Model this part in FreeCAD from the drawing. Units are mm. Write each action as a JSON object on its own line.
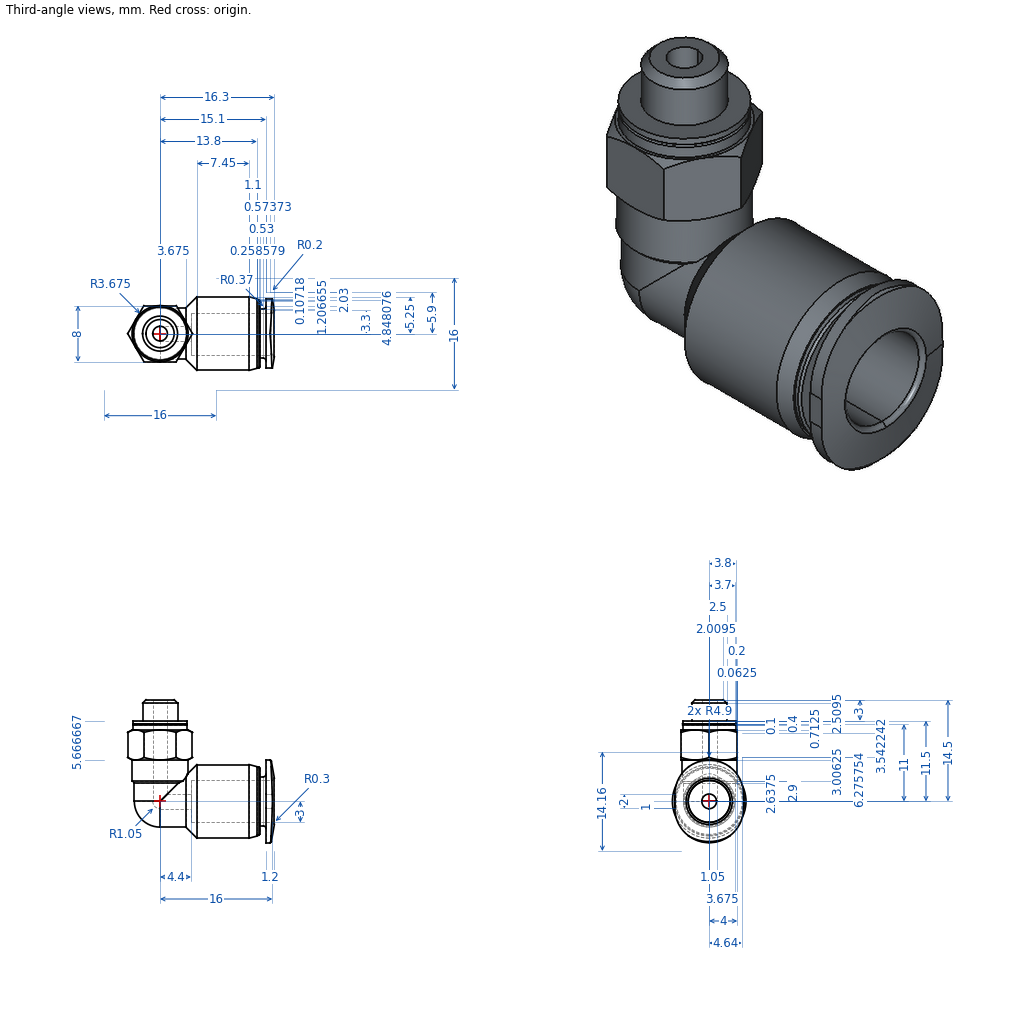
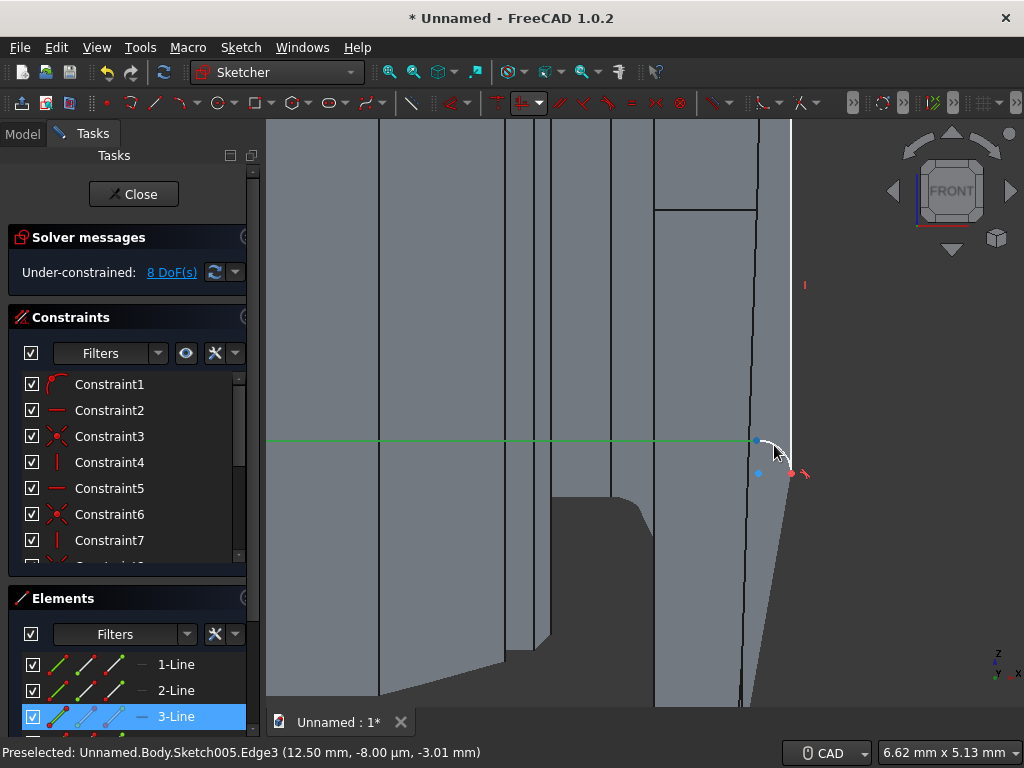
{"action": "left_click", "coordinate": [772, 443]}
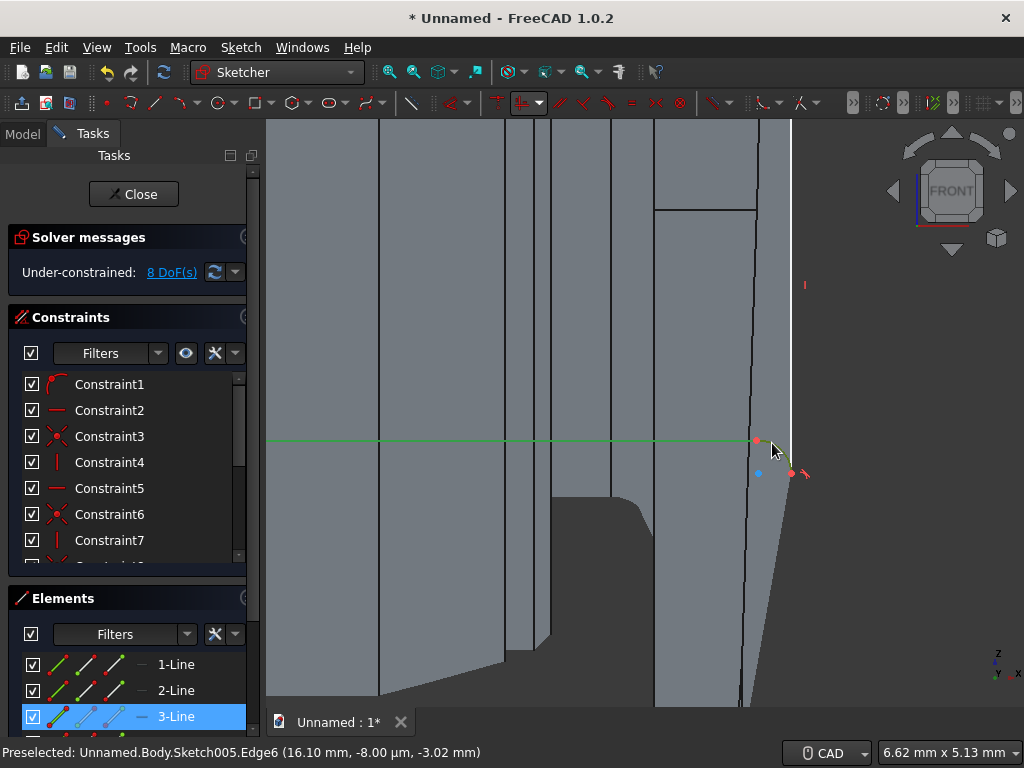
{"action": "left_click", "coordinate": [608, 104]}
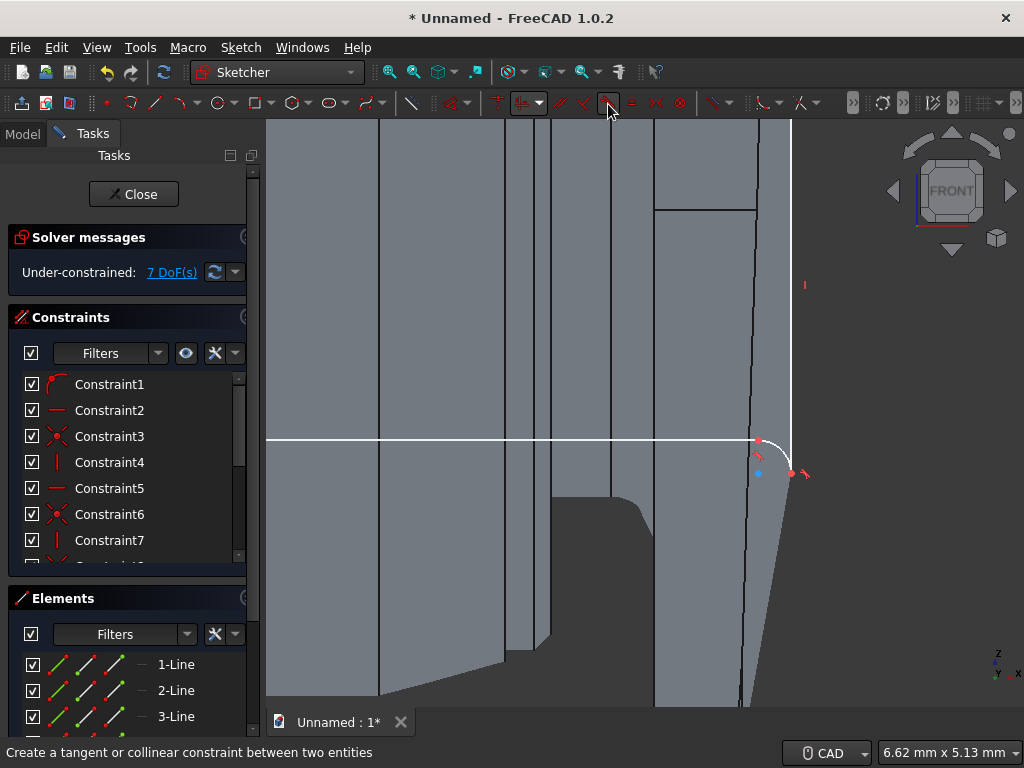
{"action": "scroll", "coordinate": [774, 445], "scroll_direction": "down", "scroll_amount": 8}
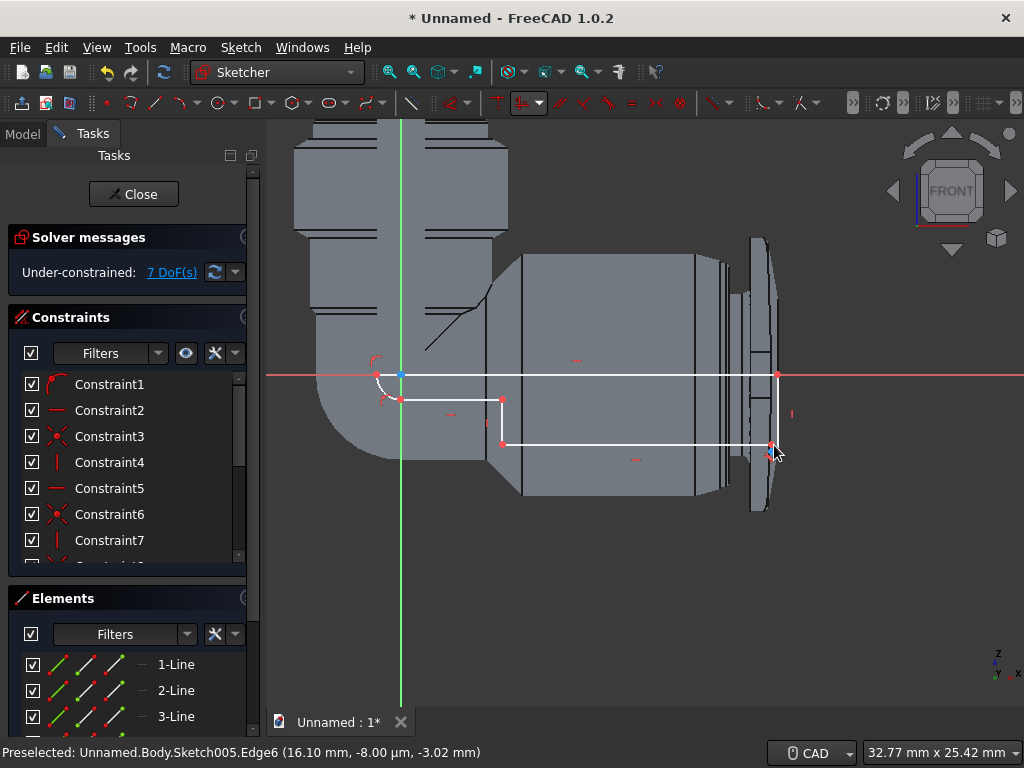
{"action": "left_click", "coordinate": [472, 400]}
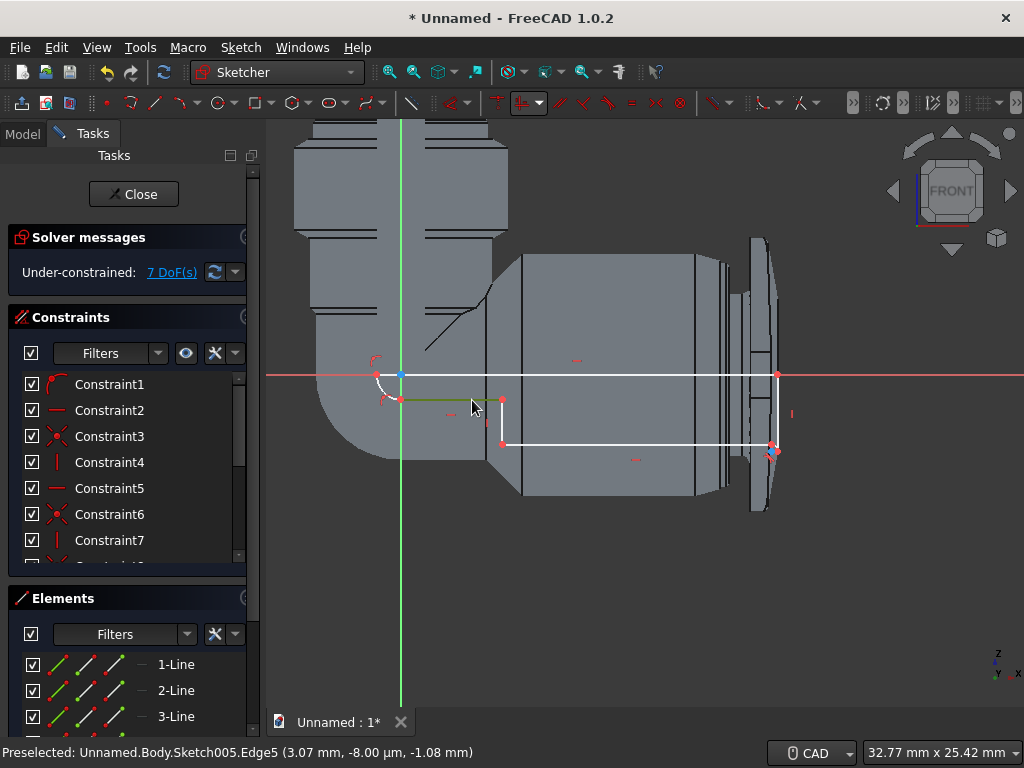
{"action": "scroll", "coordinate": [379, 386], "scroll_direction": "up", "scroll_amount": 2}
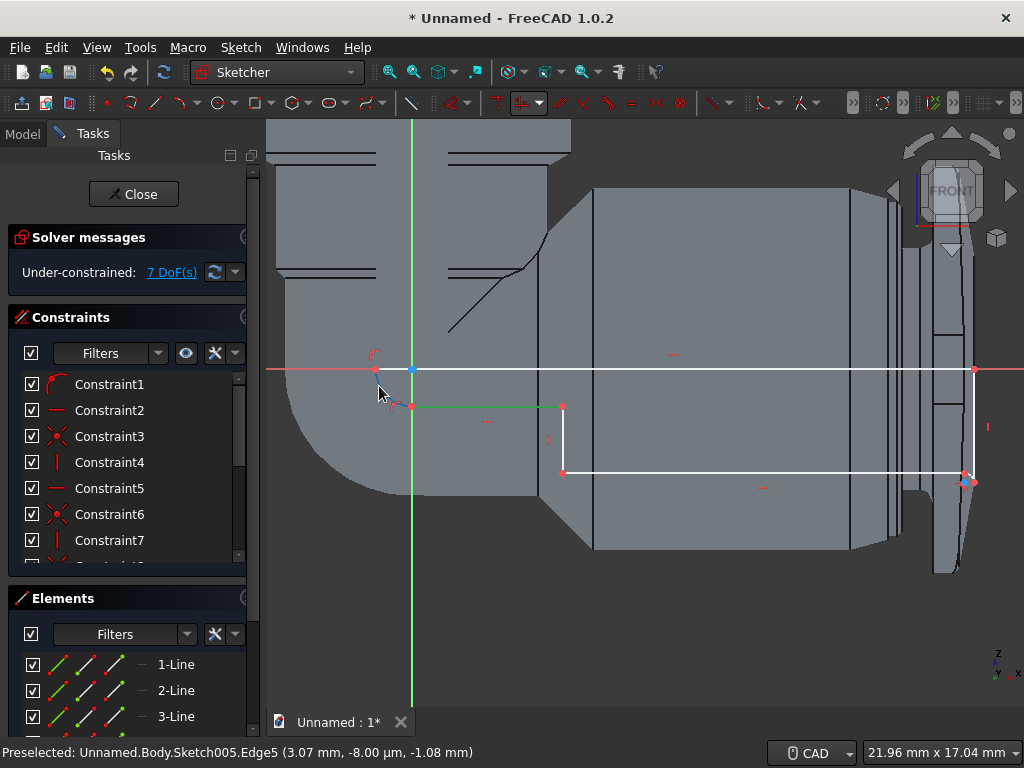
{"action": "left_click", "coordinate": [380, 386]}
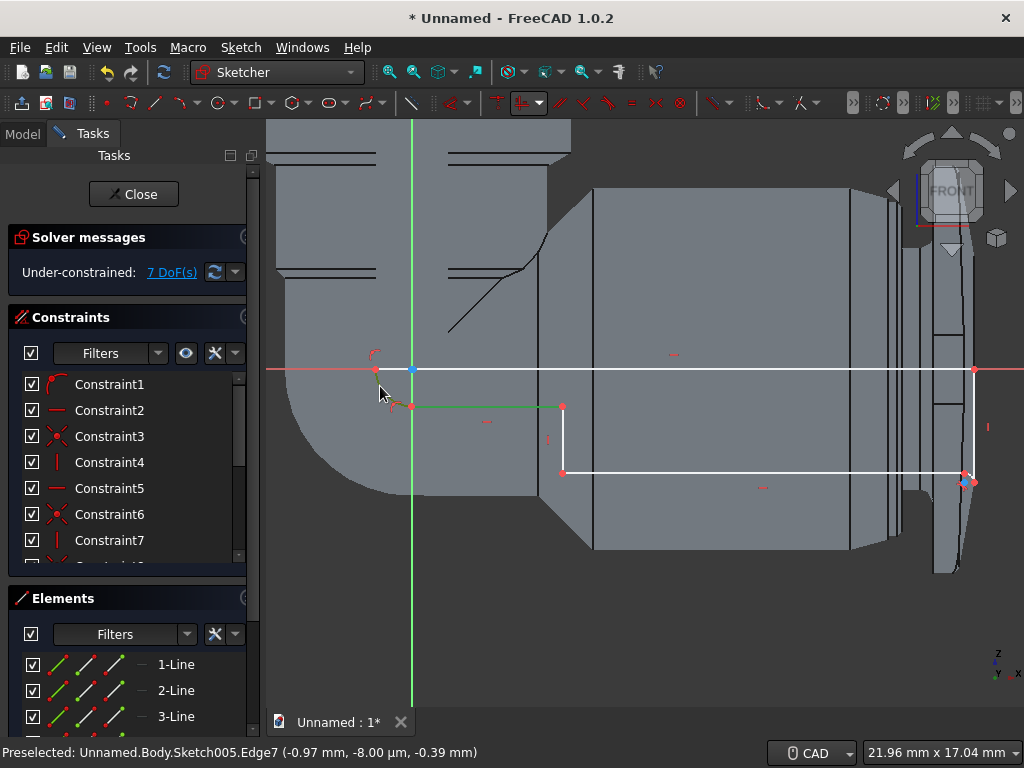
{"action": "left_click", "coordinate": [608, 104]}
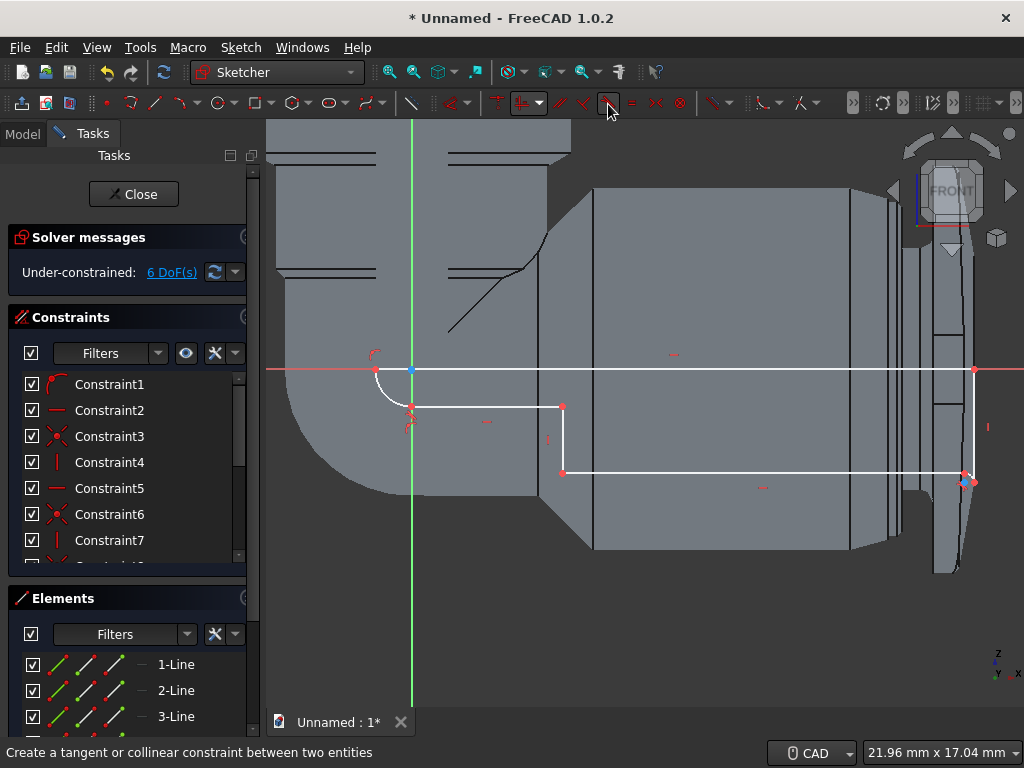
{"action": "left_click", "coordinate": [412, 371]}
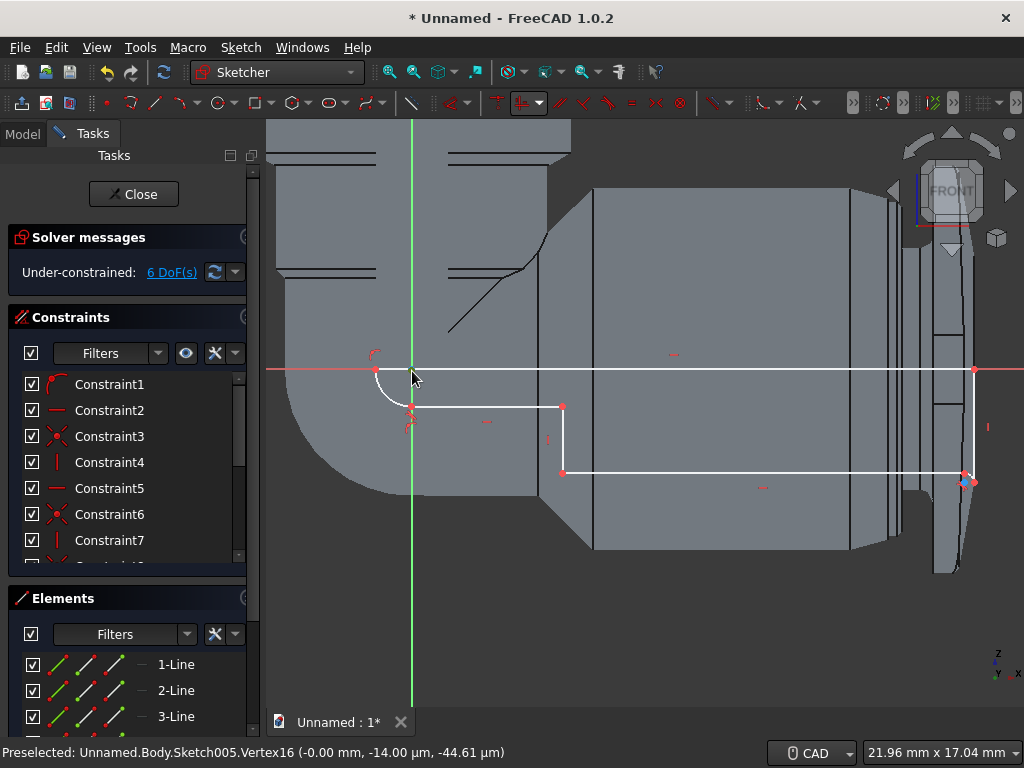
{"action": "left_click", "coordinate": [334, 369]}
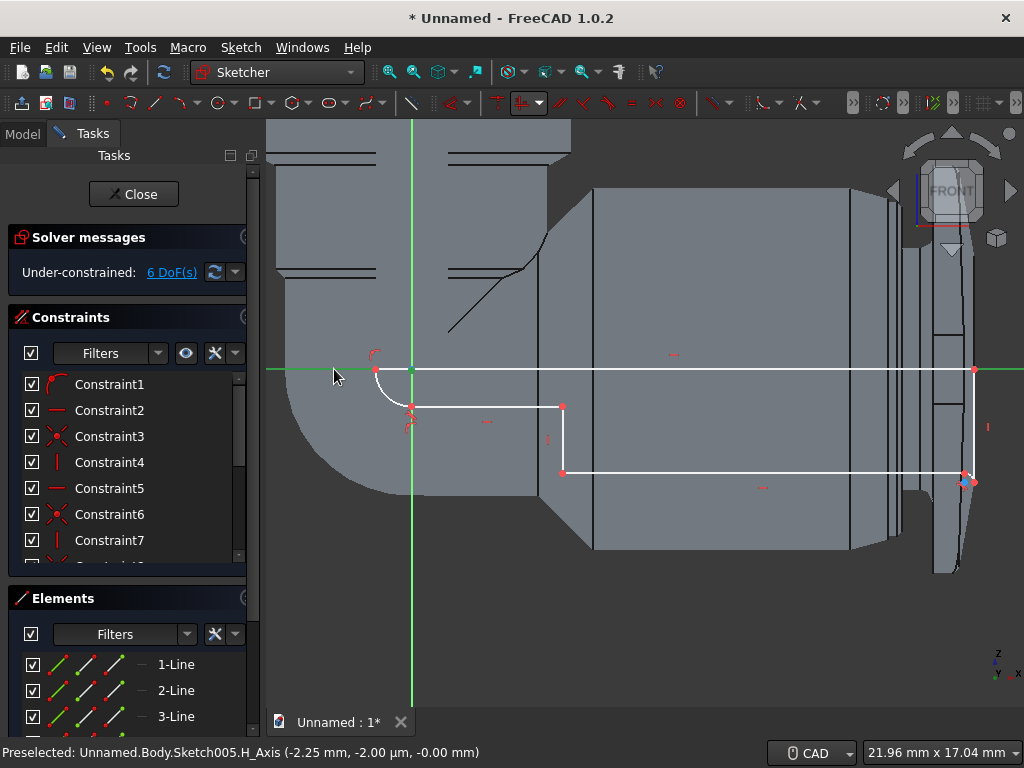
{"action": "left_click", "coordinate": [498, 104]}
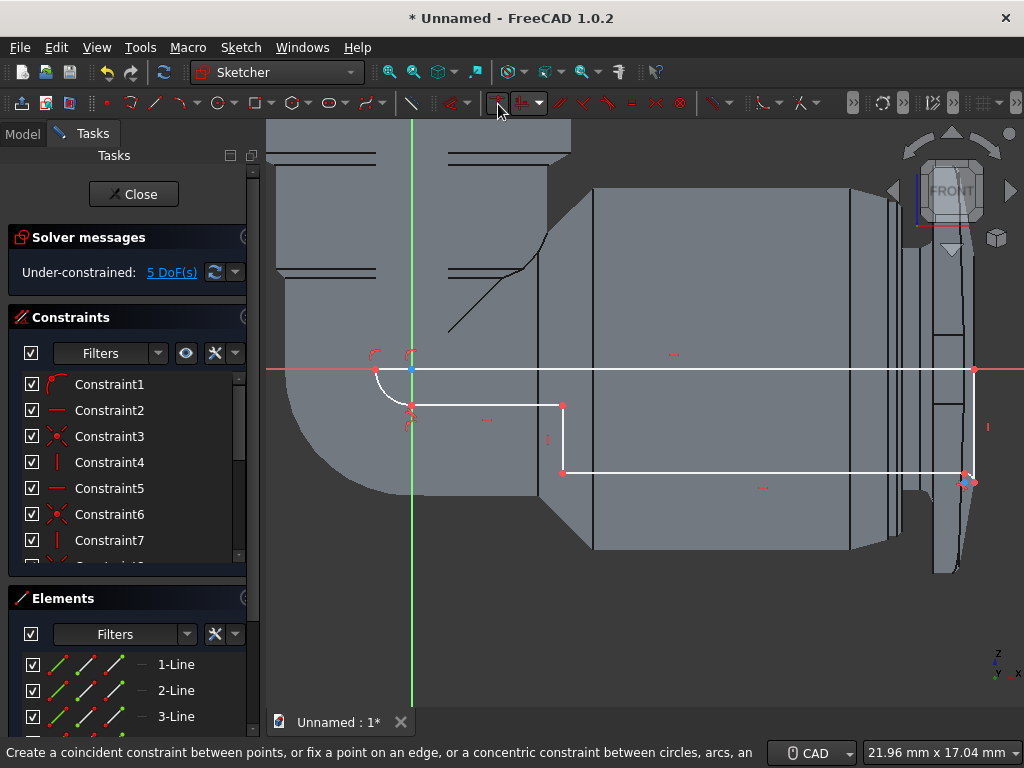
{"action": "left_click", "coordinate": [450, 104]}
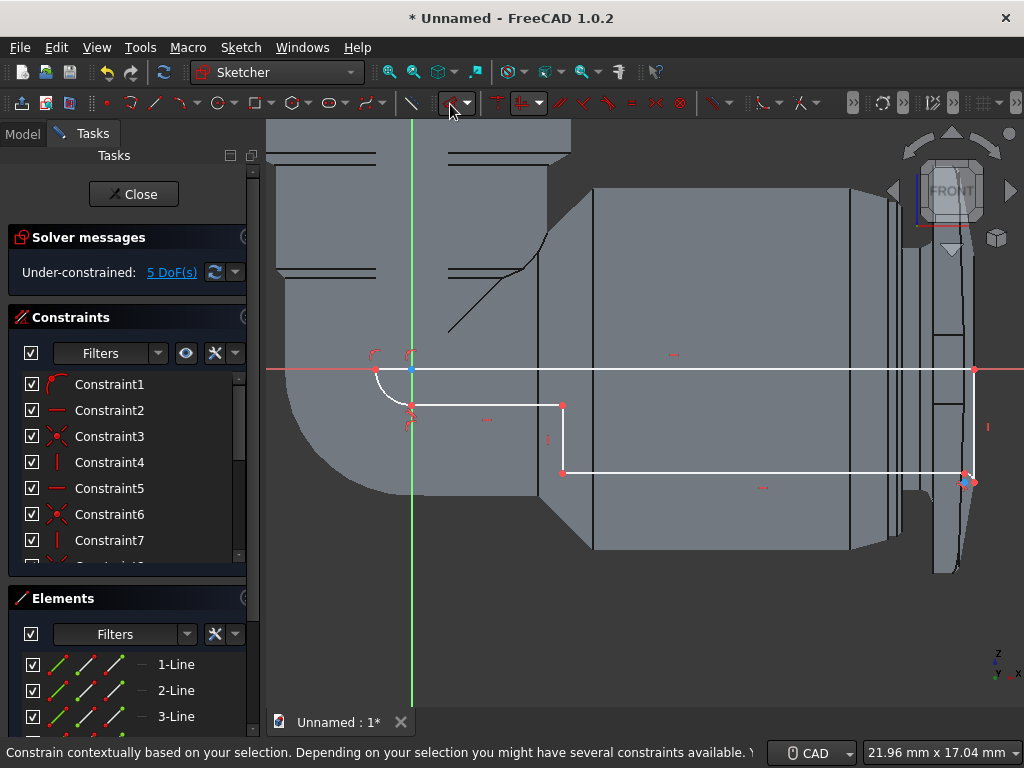
{"action": "scroll", "coordinate": [377, 386], "scroll_direction": "down", "scroll_amount": 2}